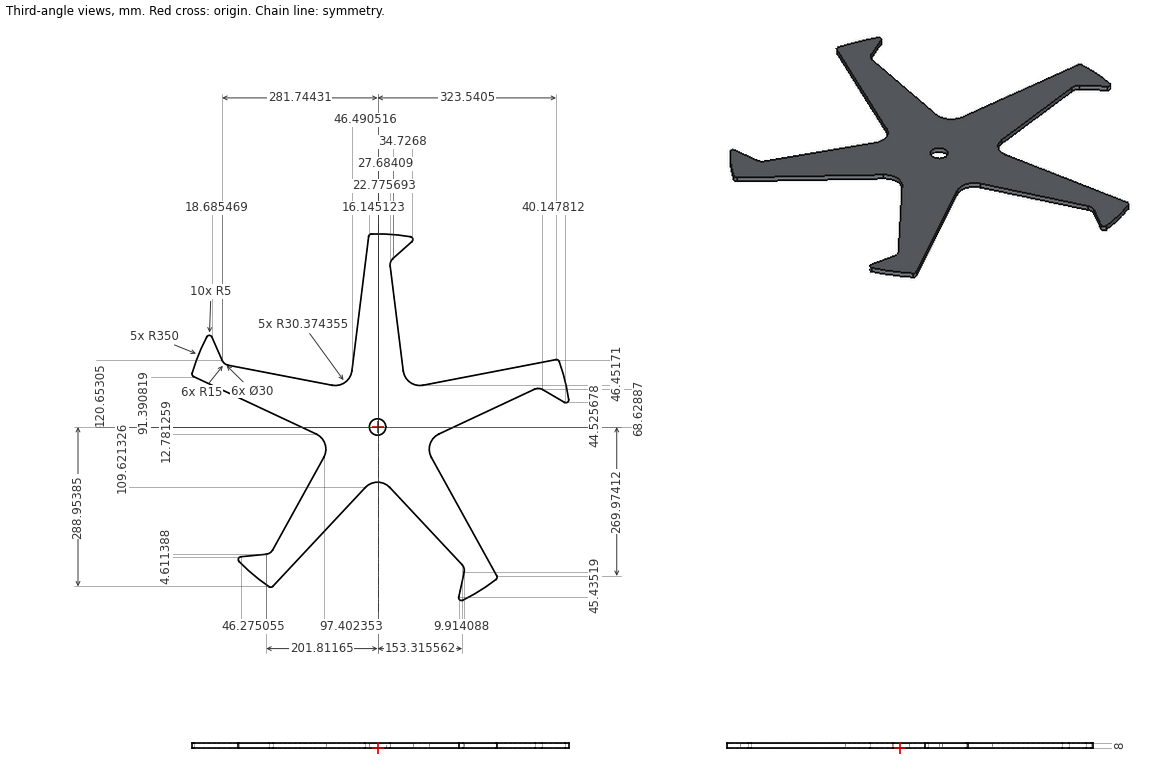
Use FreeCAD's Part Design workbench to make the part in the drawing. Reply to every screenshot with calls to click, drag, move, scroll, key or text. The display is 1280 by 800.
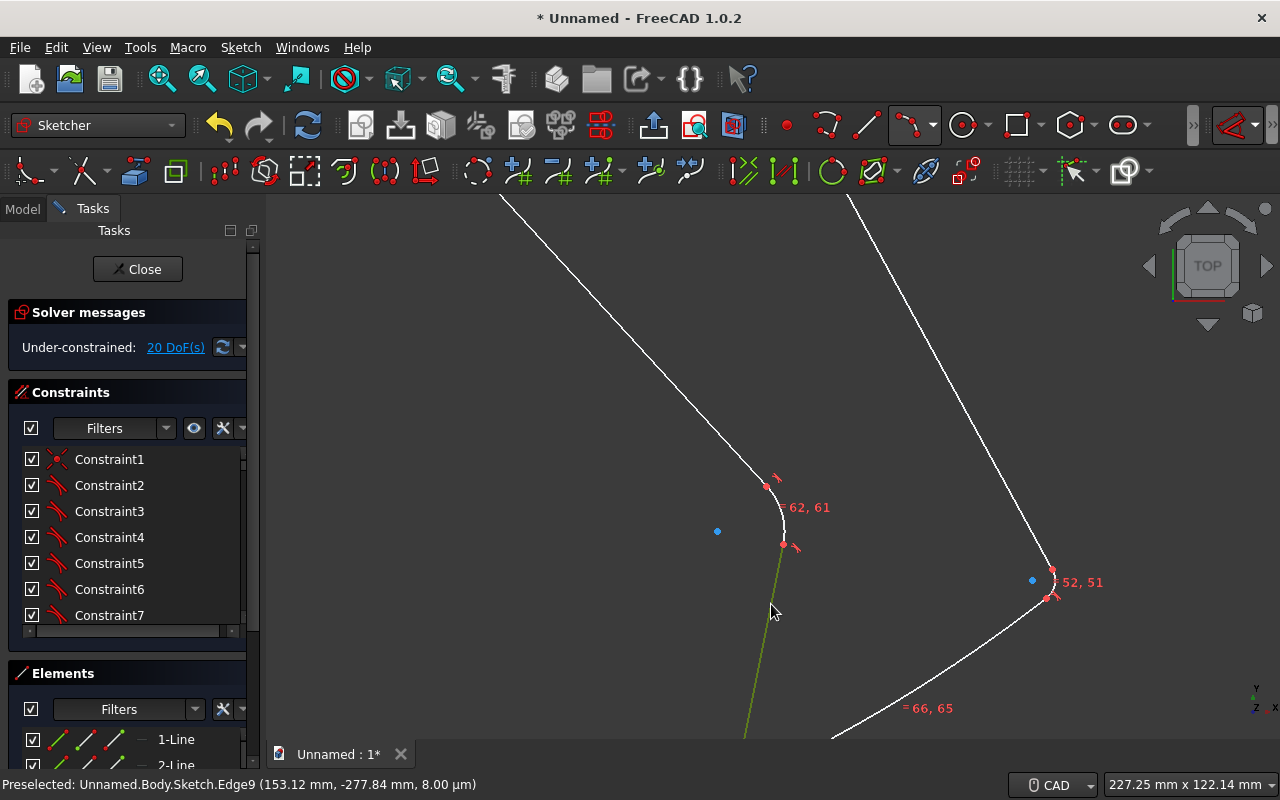
click(1258, 126)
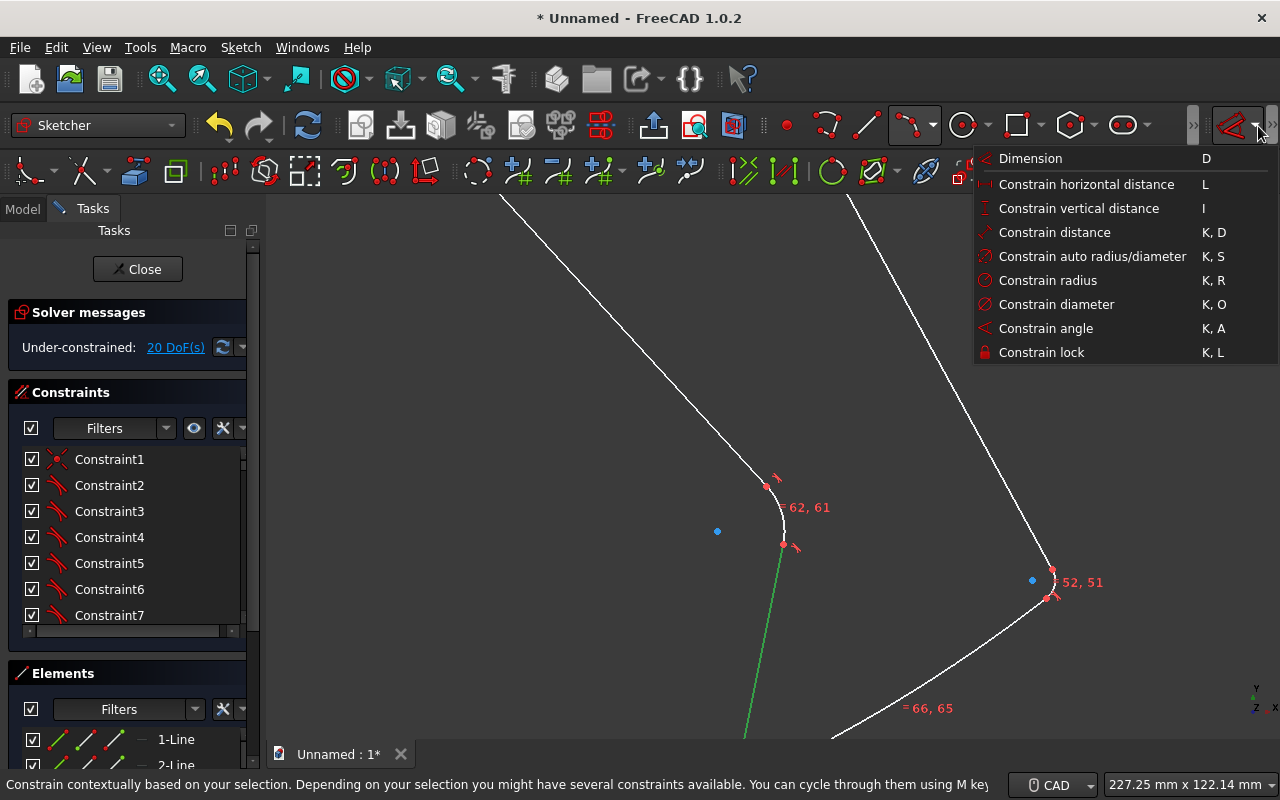
click(1126, 184)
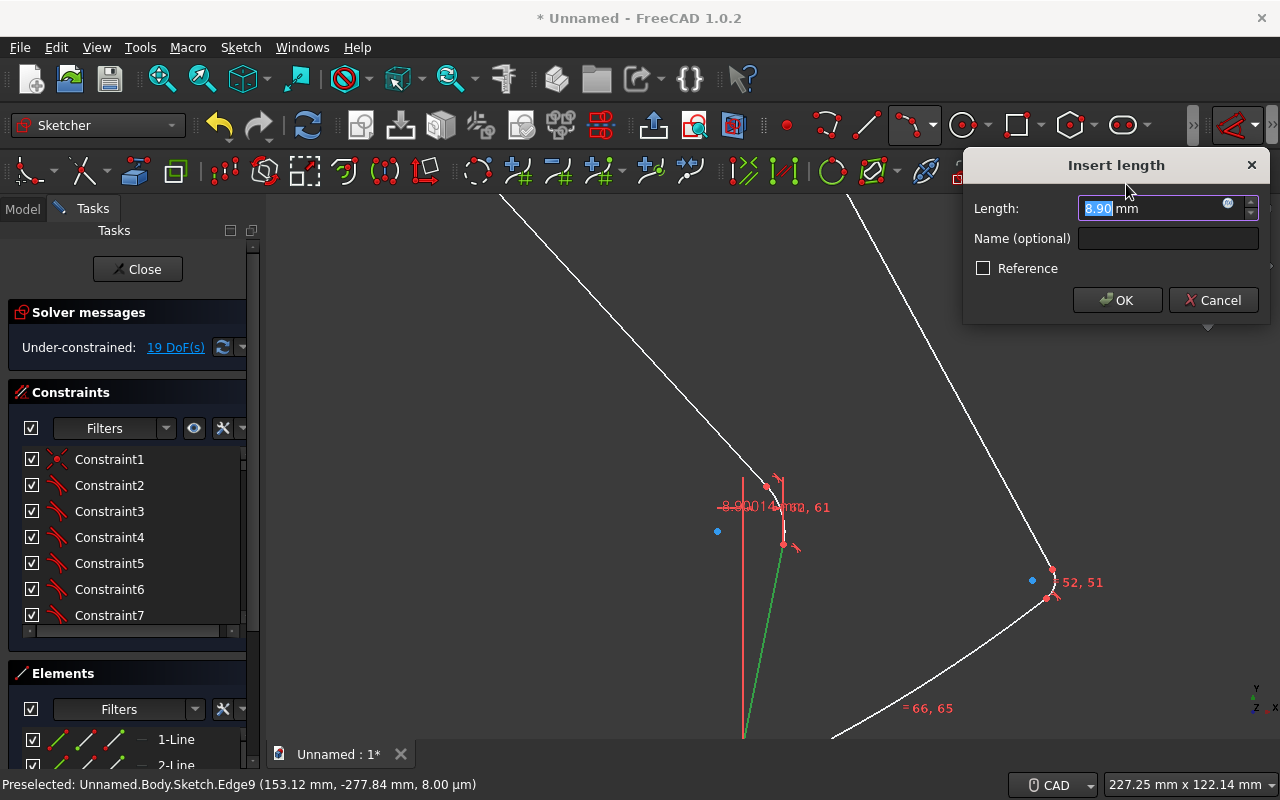
text(9.914088)
key(Return)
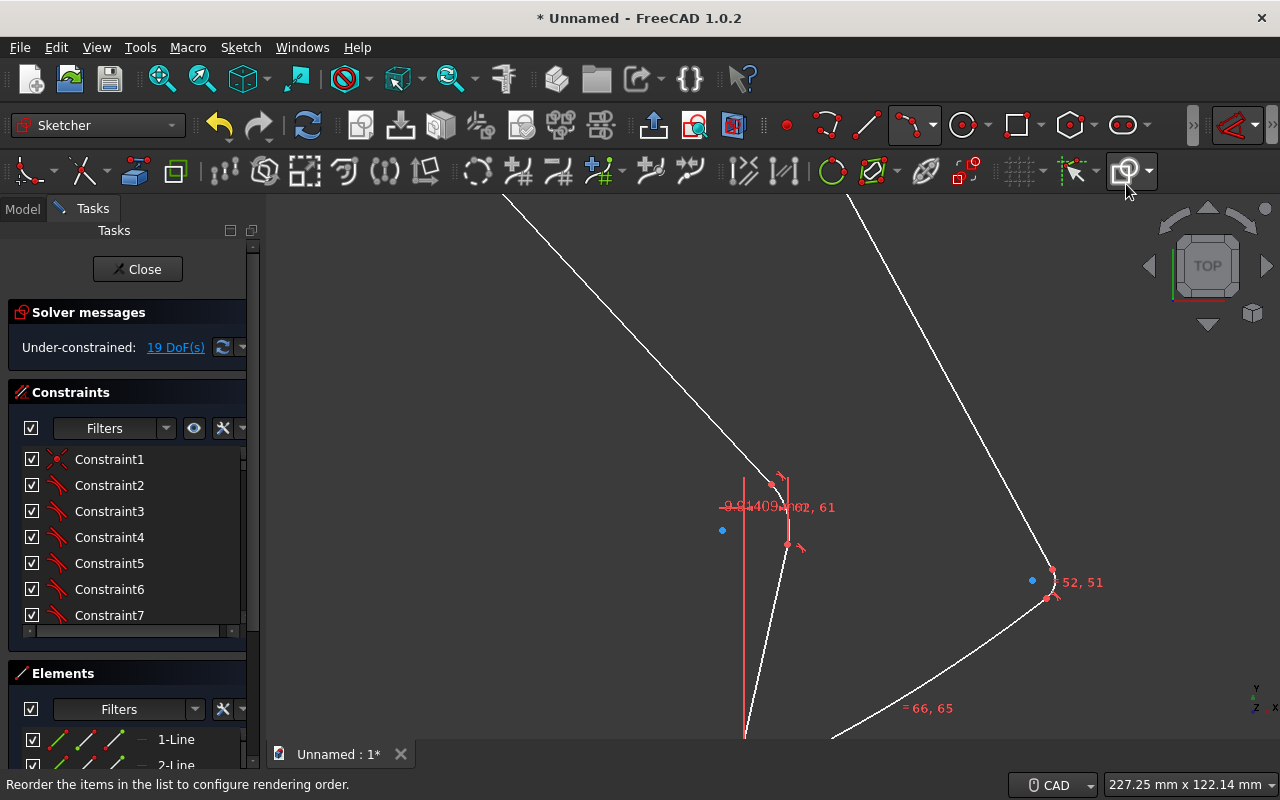
scroll(778, 614, down, 11)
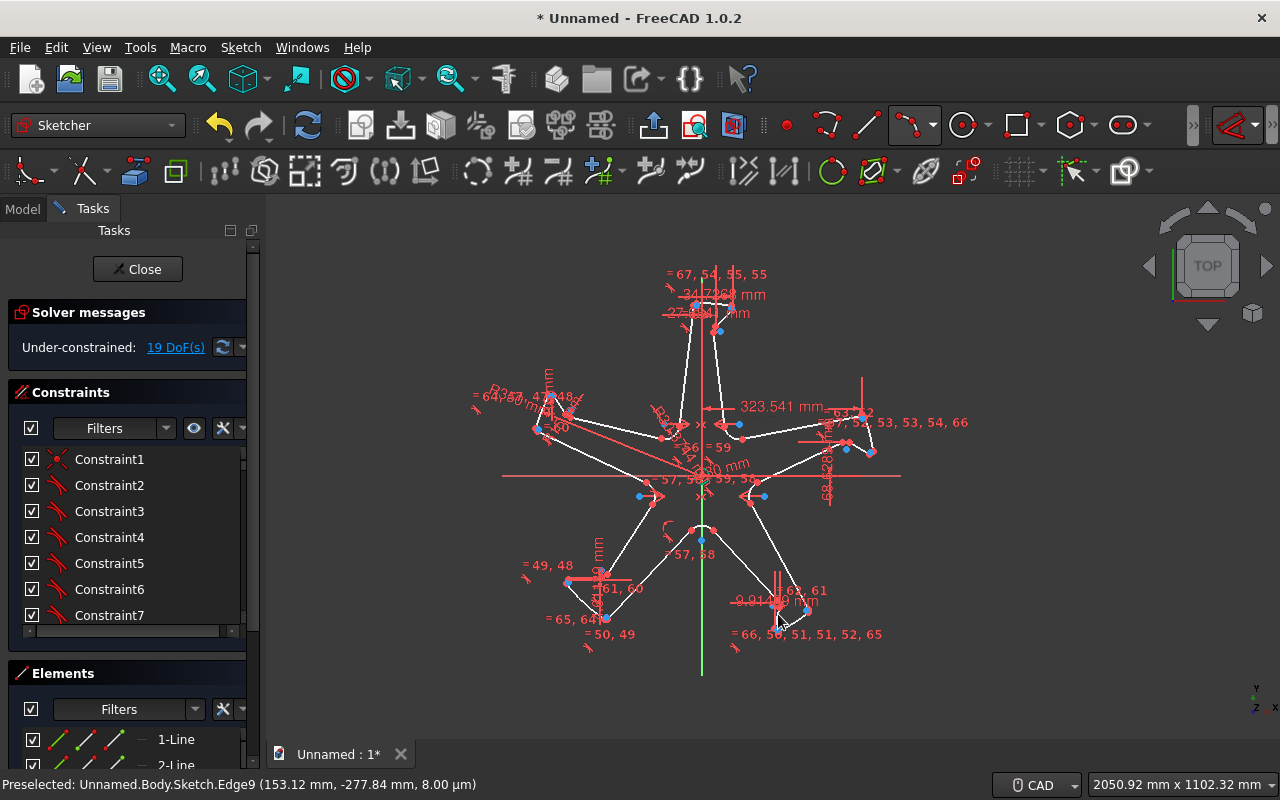
scroll(778, 614, up, 4)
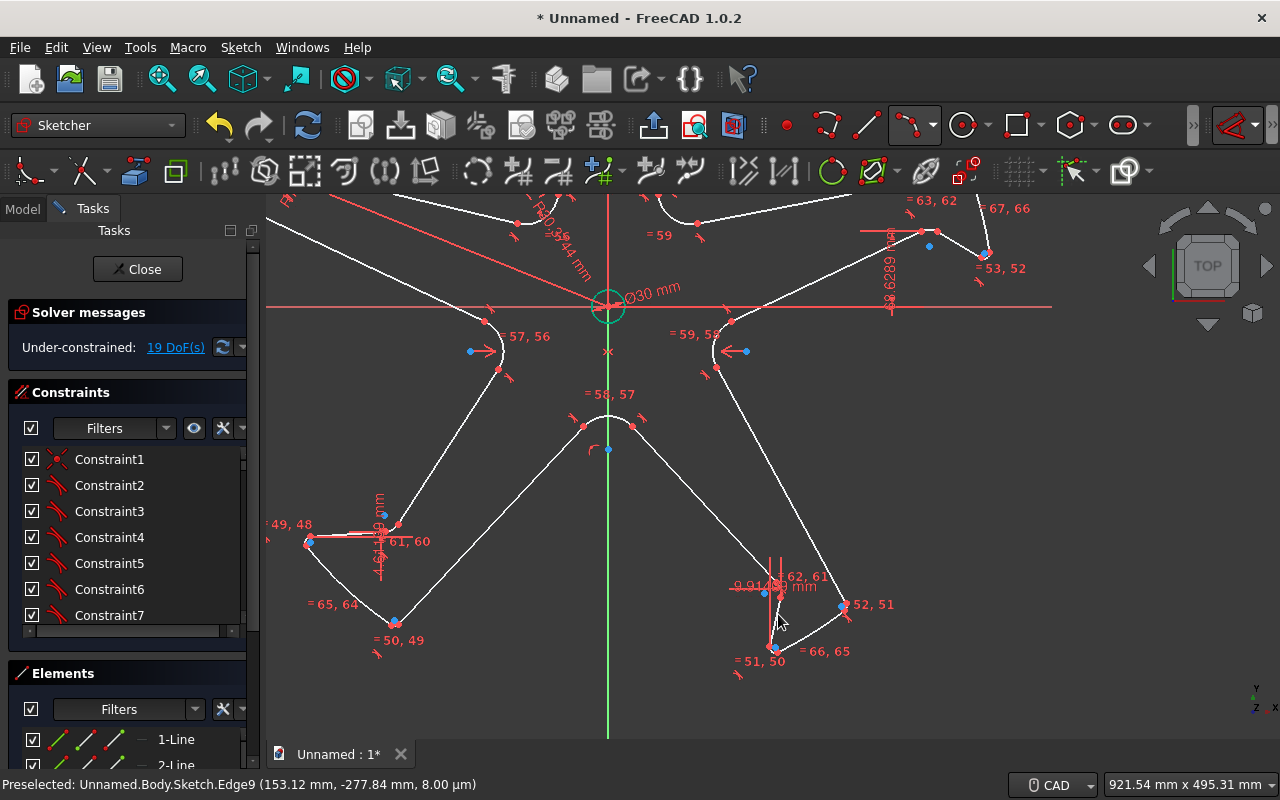
click(778, 612)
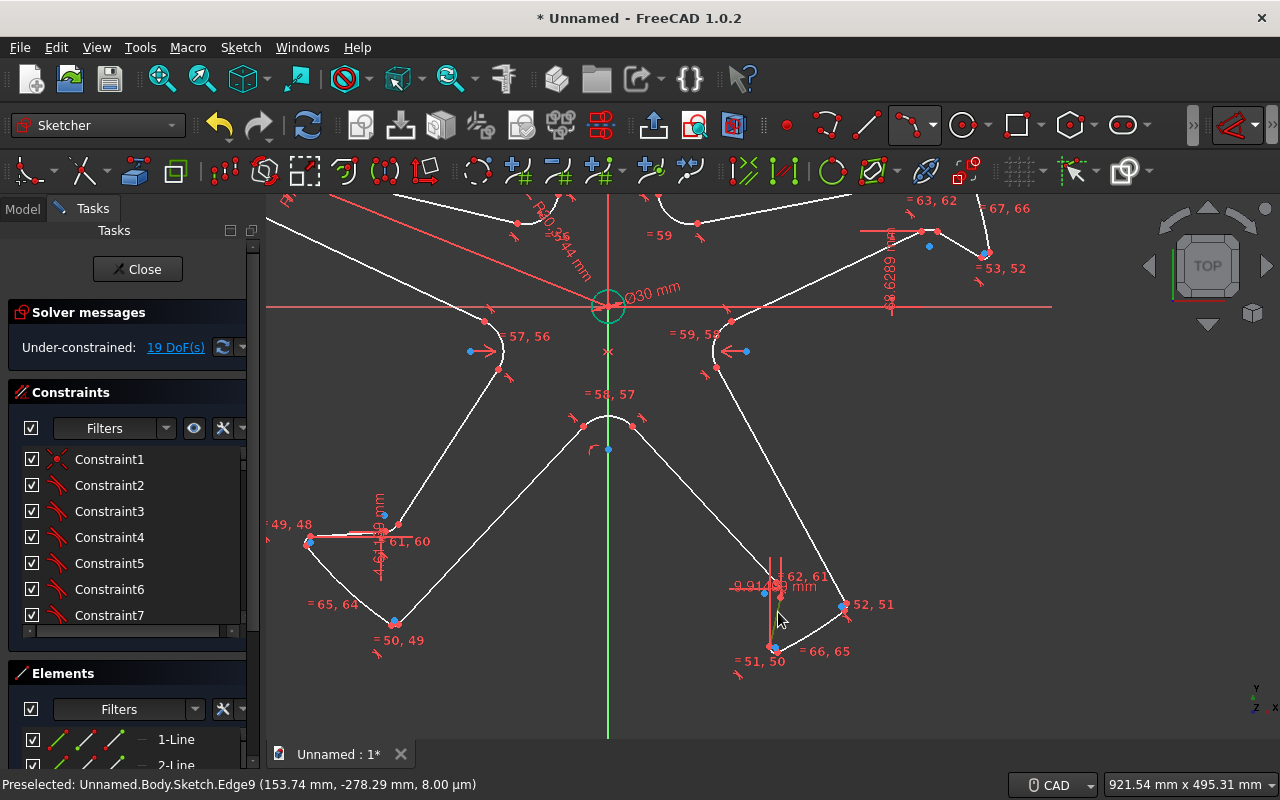
key(i)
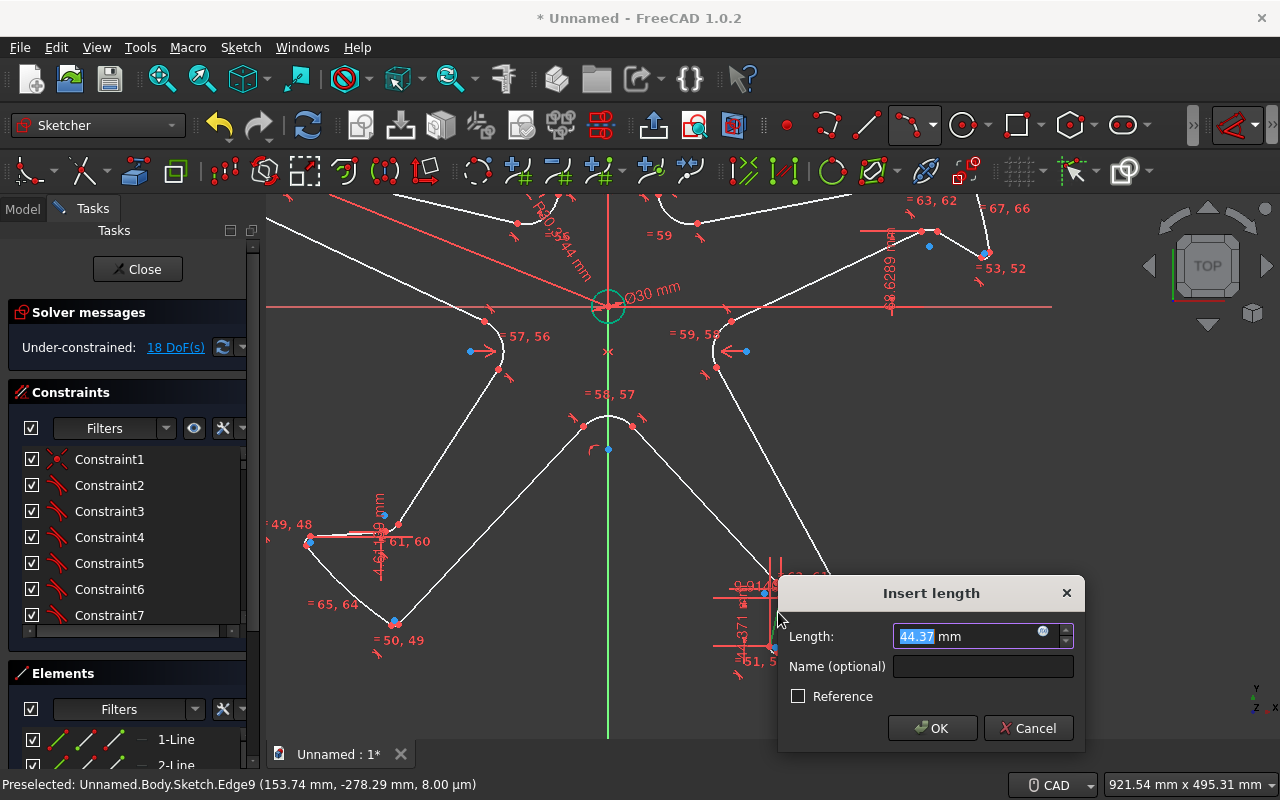
text(45.43519)
key(Return)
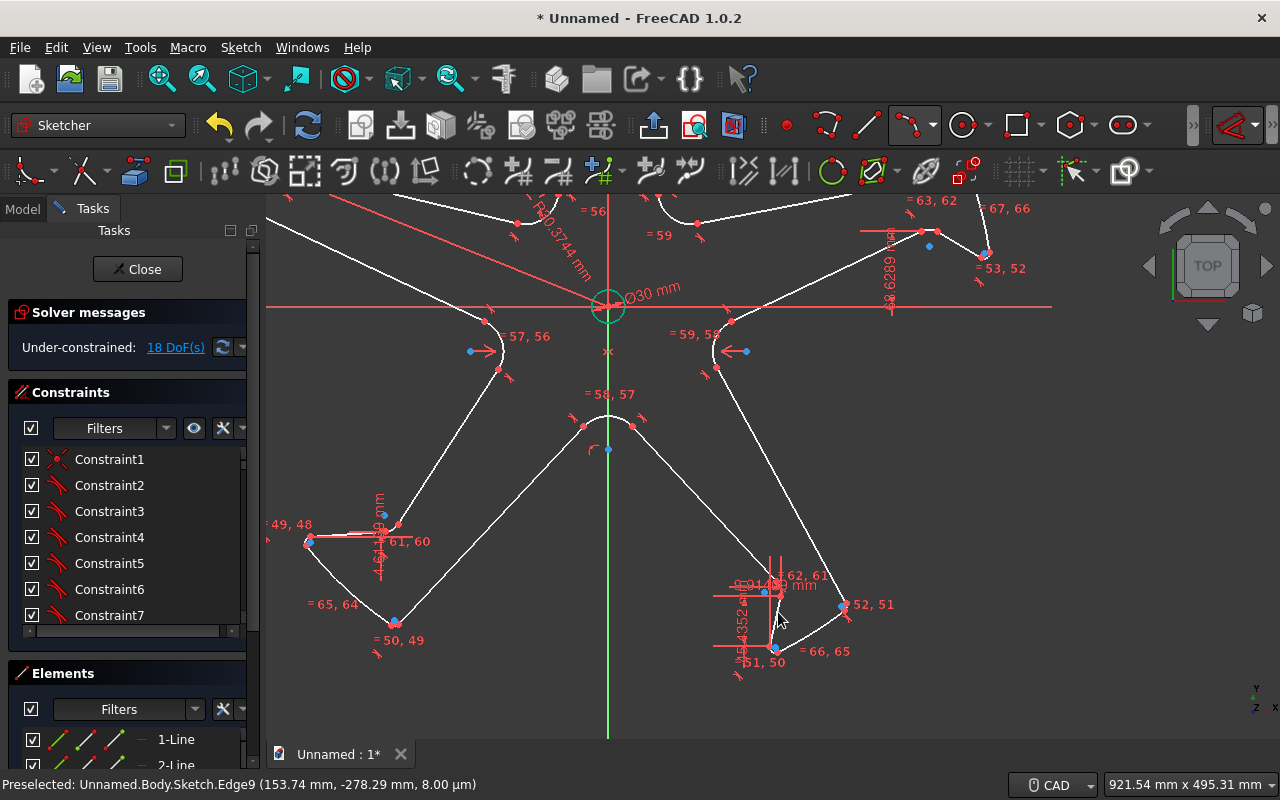
scroll(778, 613, down, 4)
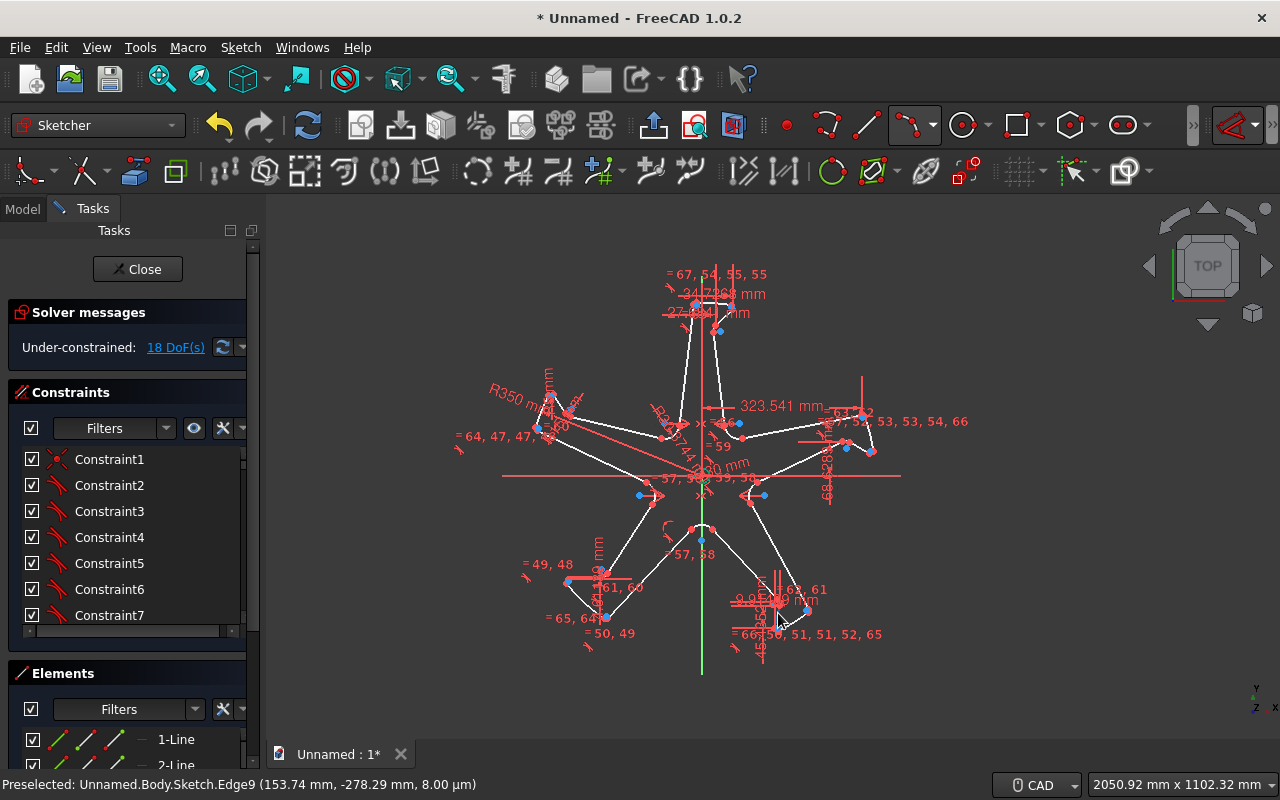
scroll(826, 422, up, 3)